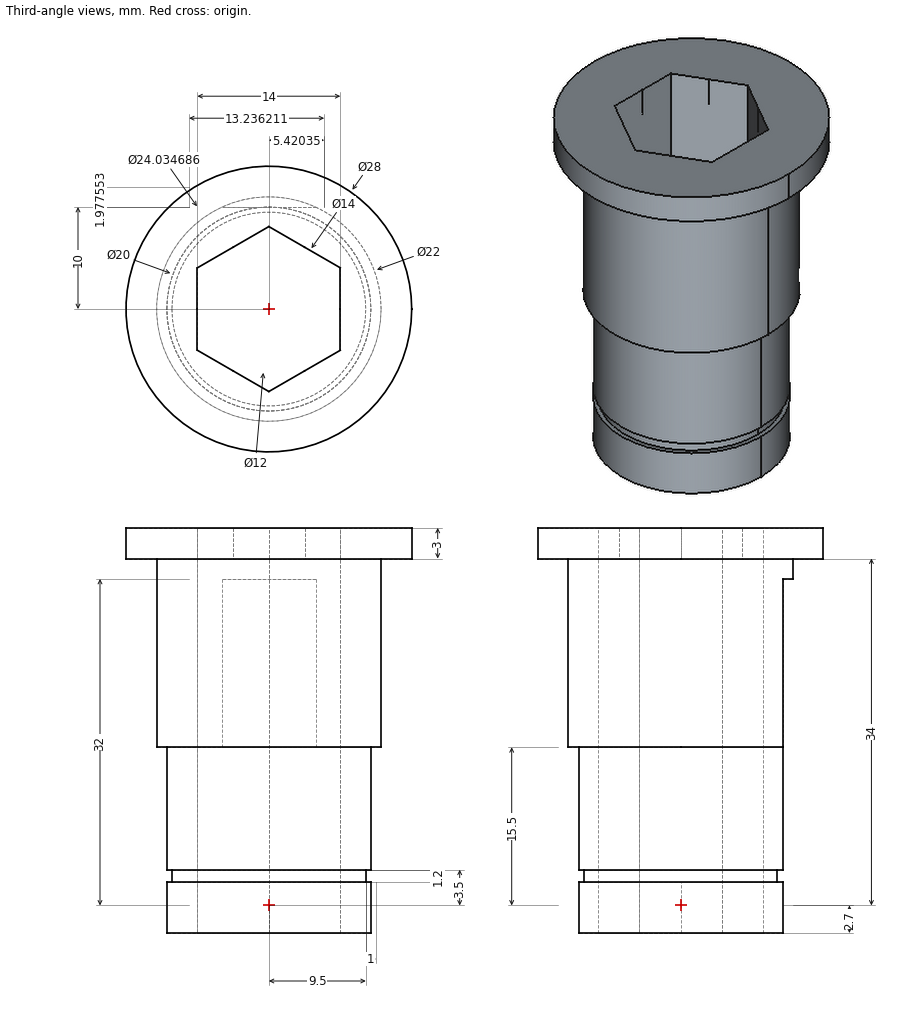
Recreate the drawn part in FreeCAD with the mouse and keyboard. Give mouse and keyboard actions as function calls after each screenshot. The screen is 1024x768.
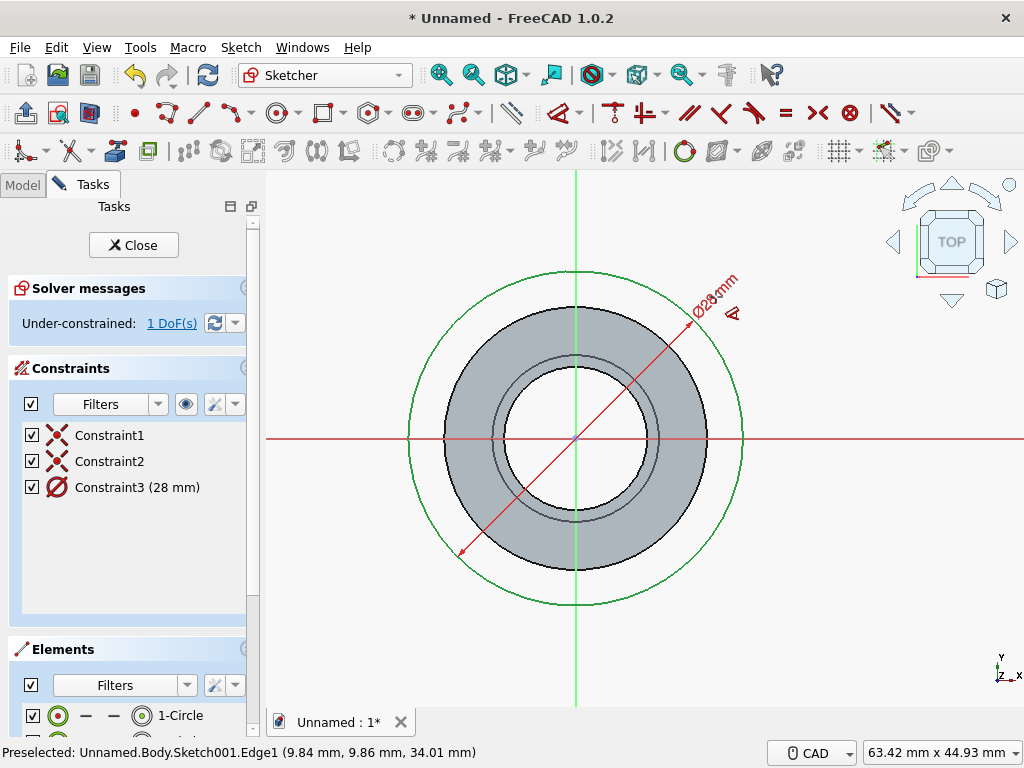
click(634, 379)
click(656, 356)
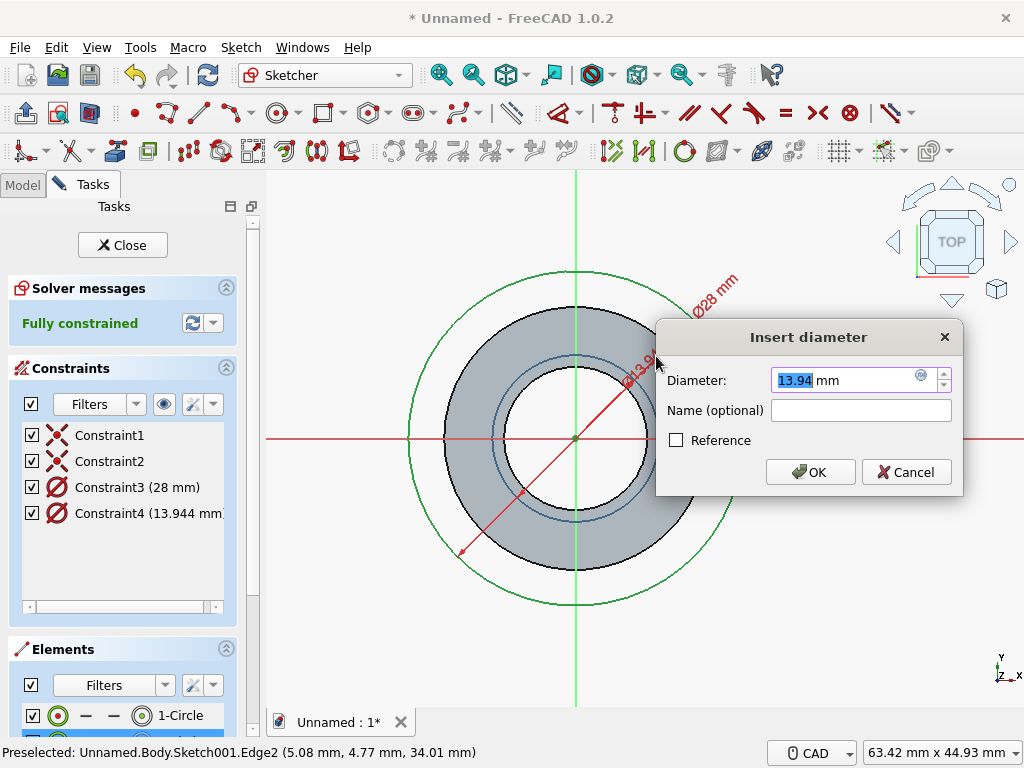
text(14)
key(Return)
key(Escape)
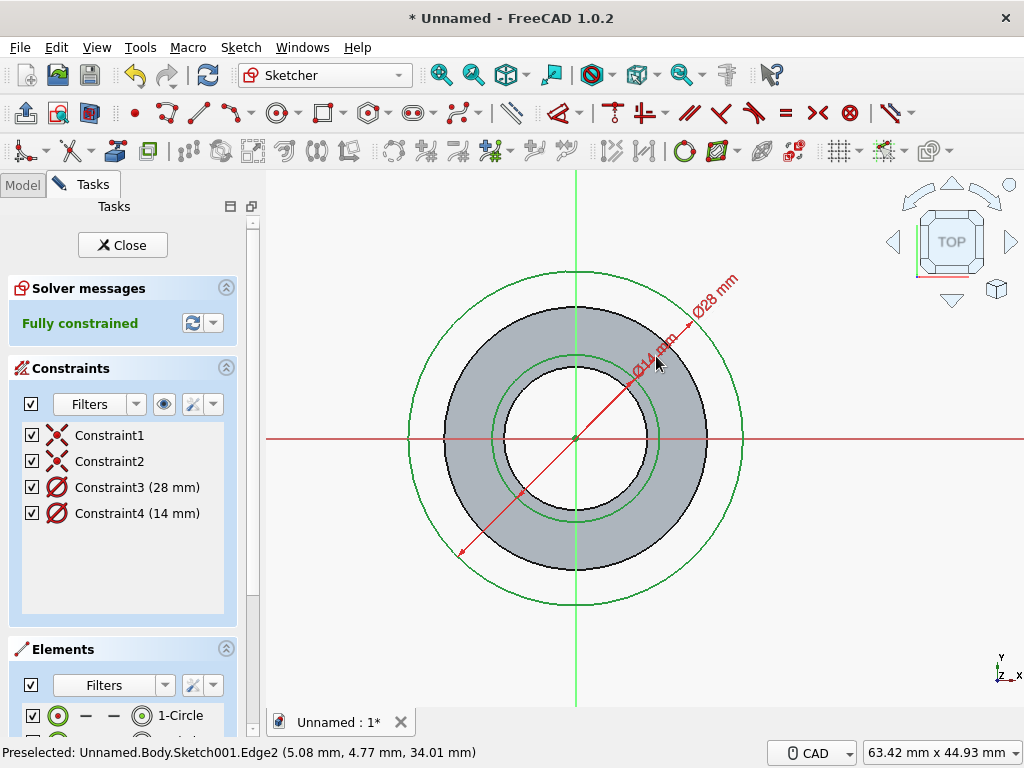
click(123, 245)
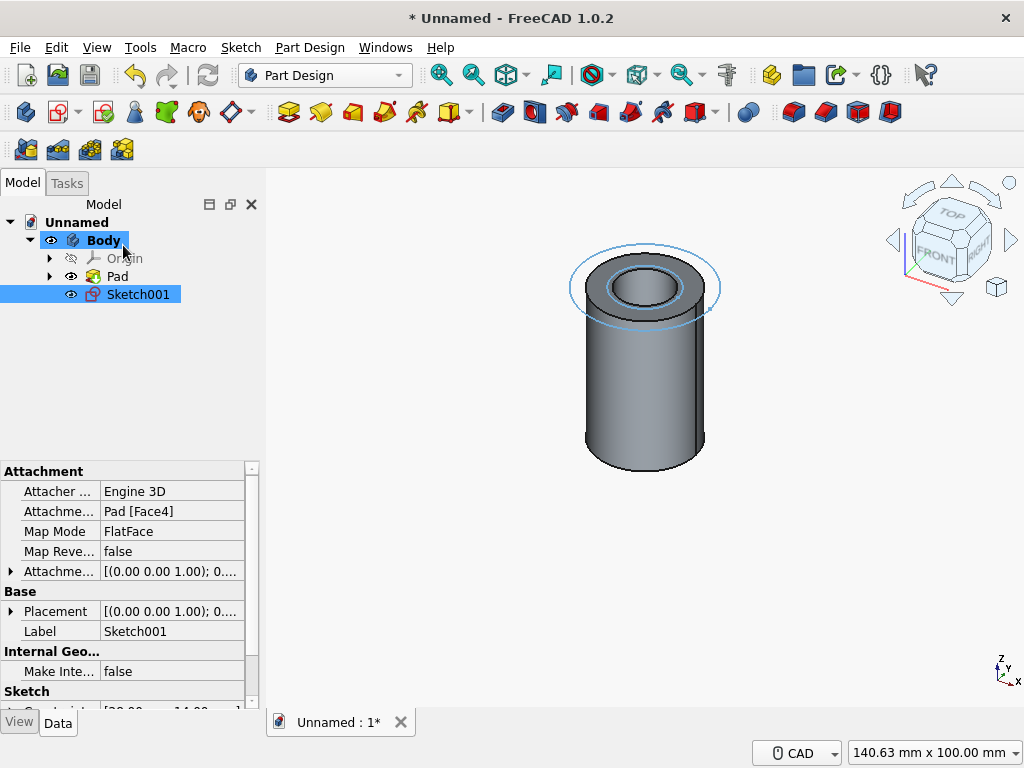
click(290, 112)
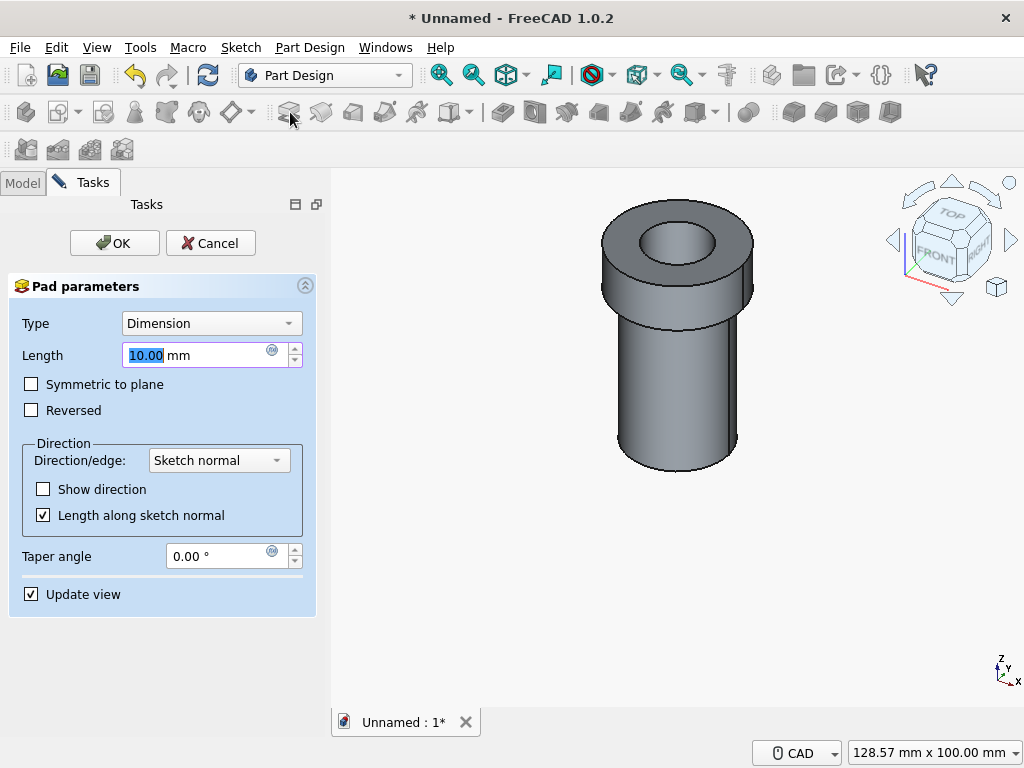
text(3)
key(Tab)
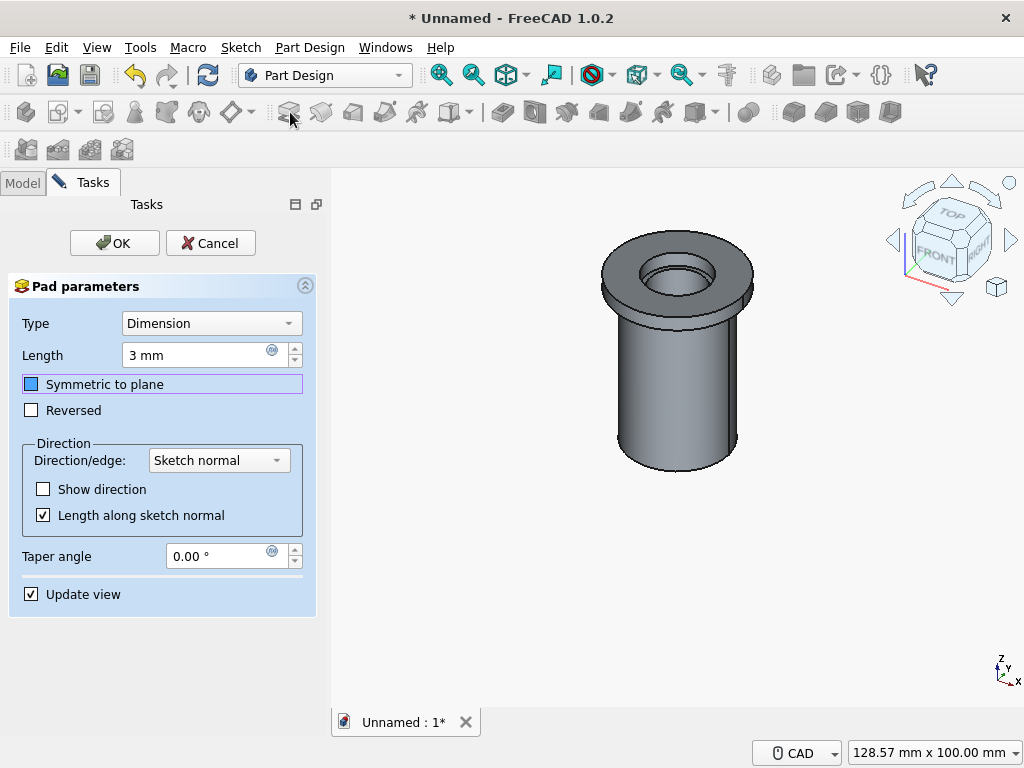
click(115, 243)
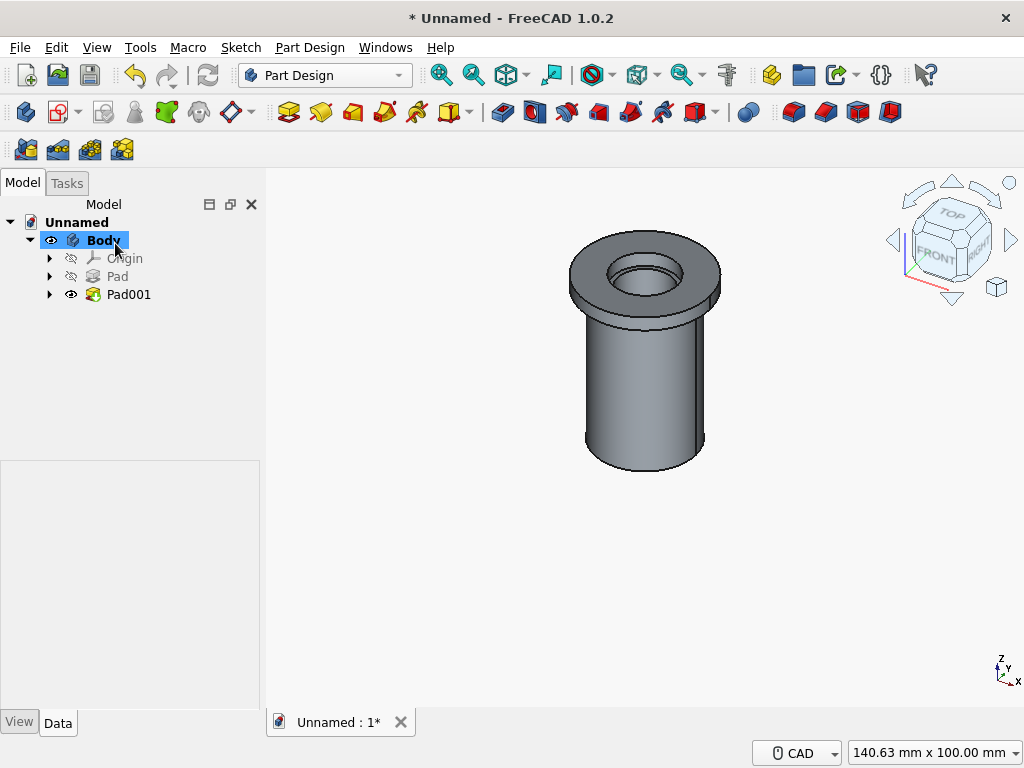
key(5)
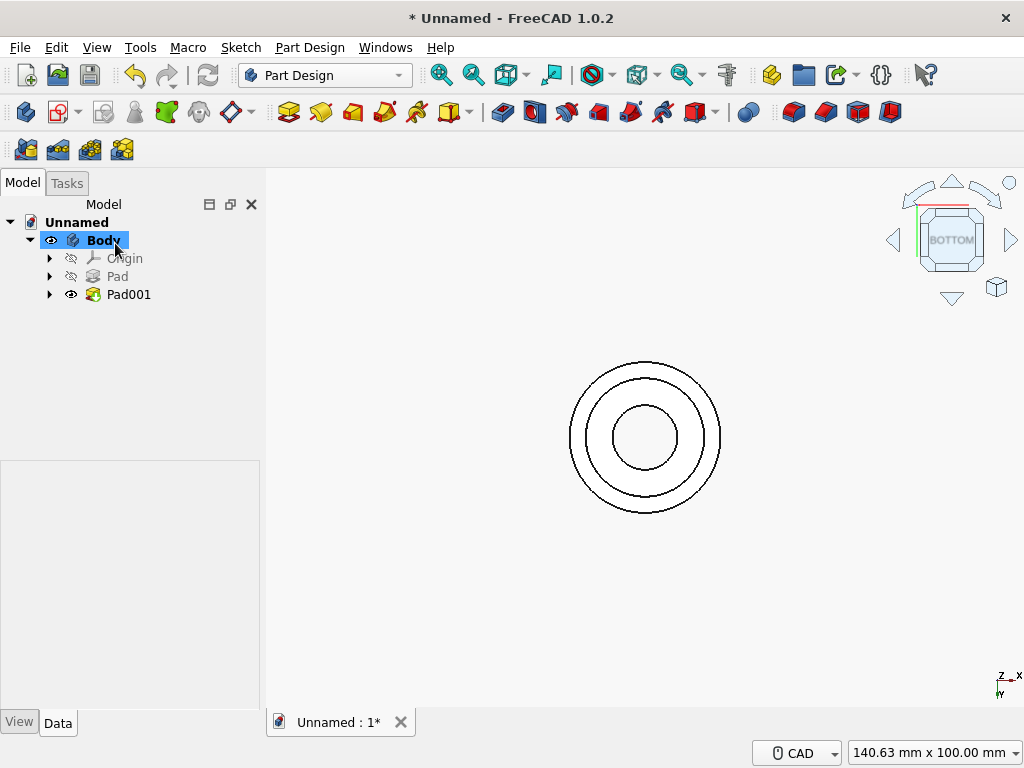
click(442, 76)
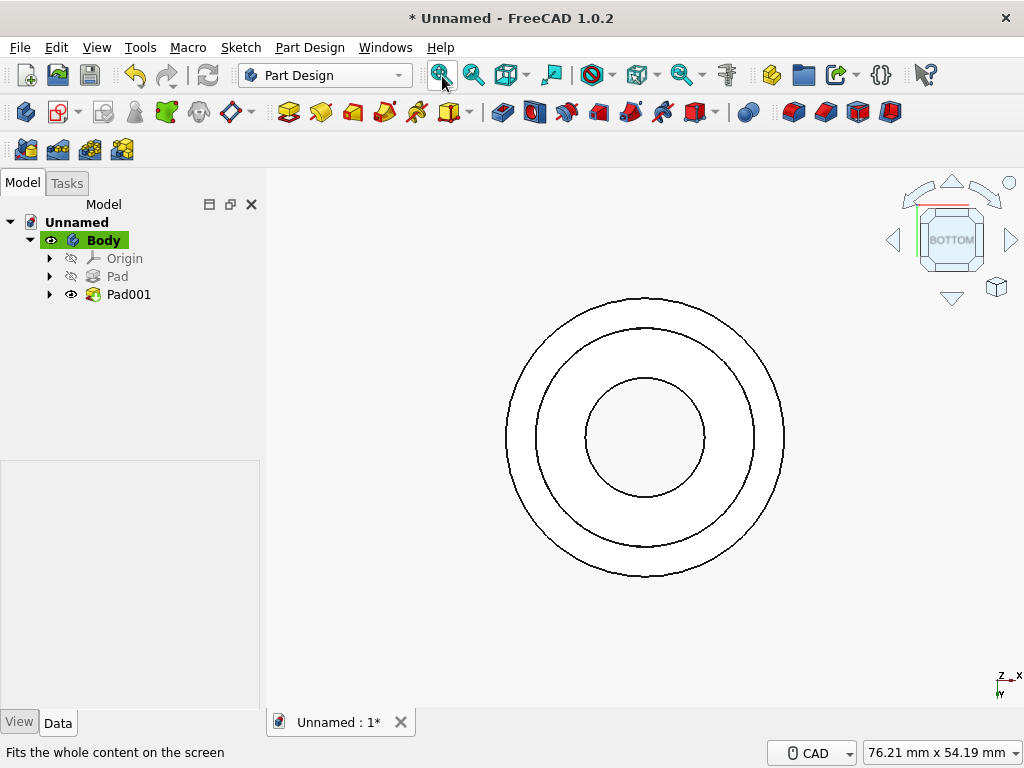
click(708, 499)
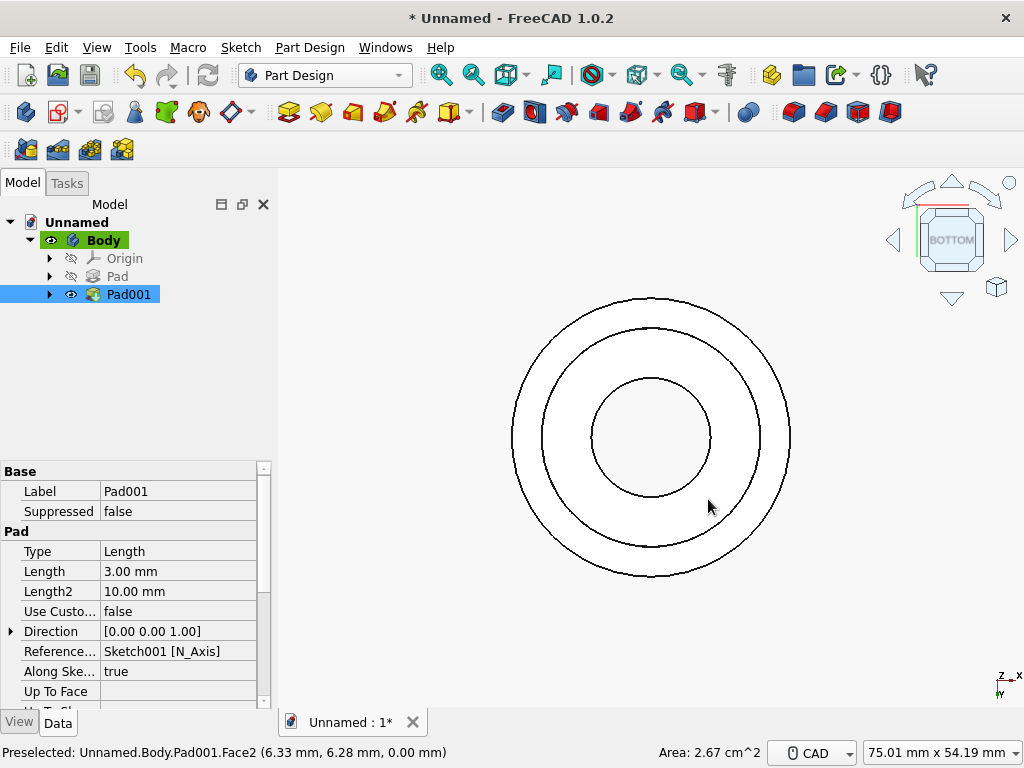
click(58, 112)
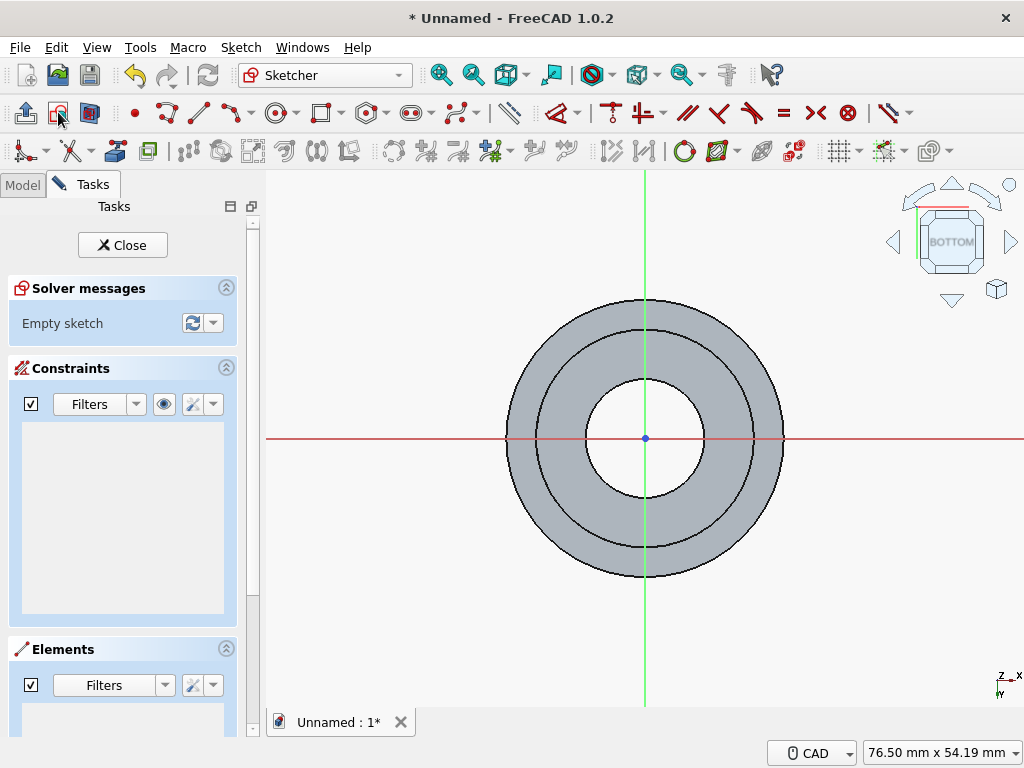
scroll(784, 439, up, 2)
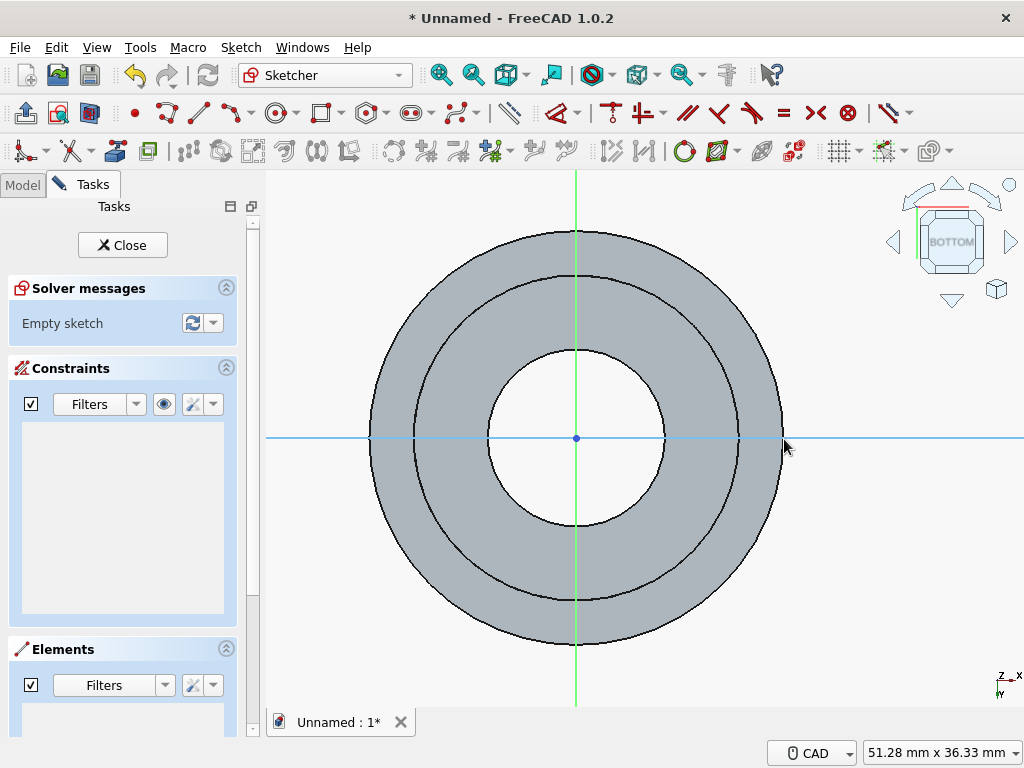
click(276, 114)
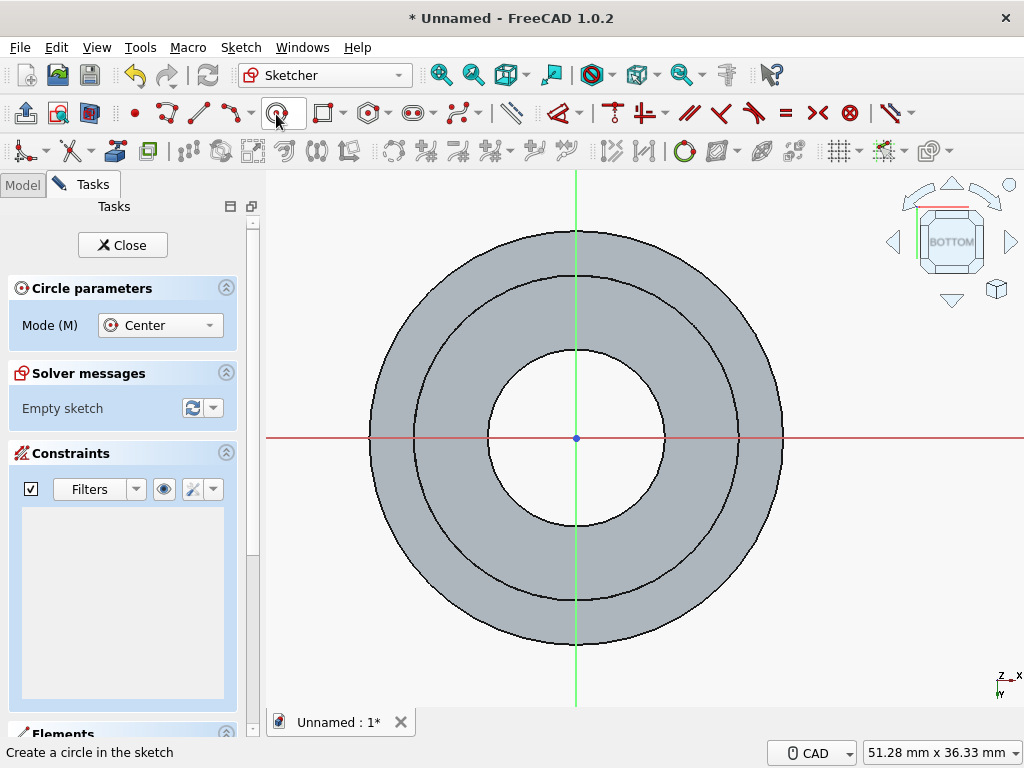
click(576, 438)
click(702, 312)